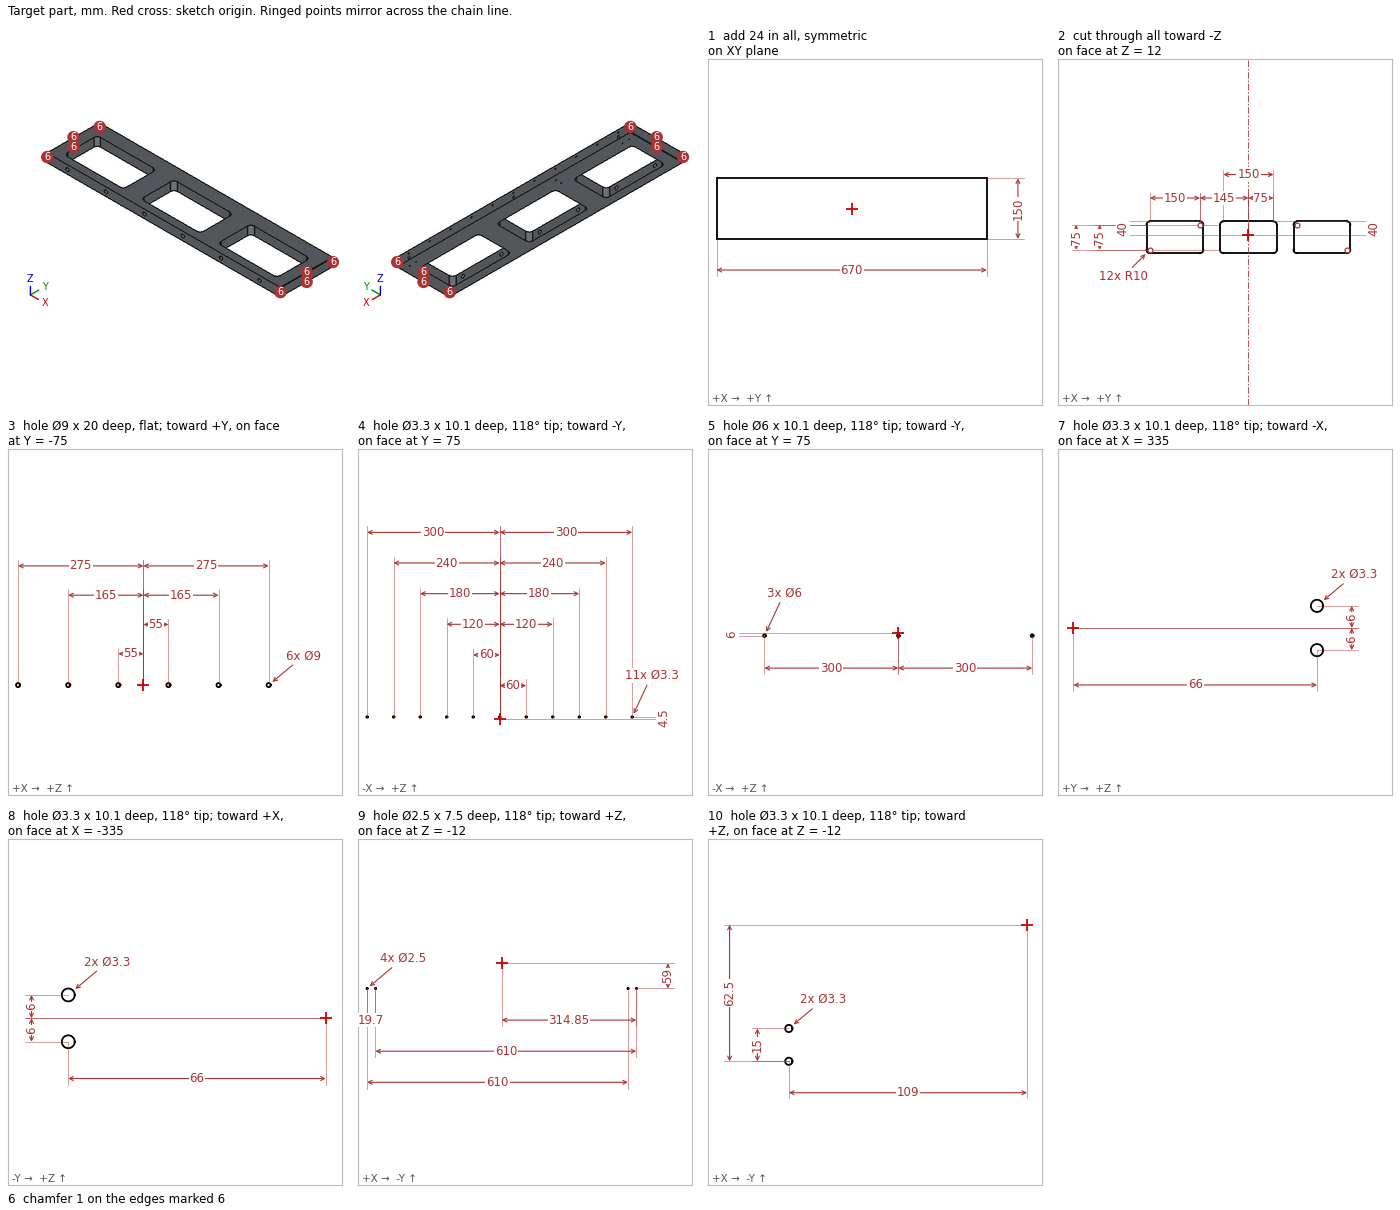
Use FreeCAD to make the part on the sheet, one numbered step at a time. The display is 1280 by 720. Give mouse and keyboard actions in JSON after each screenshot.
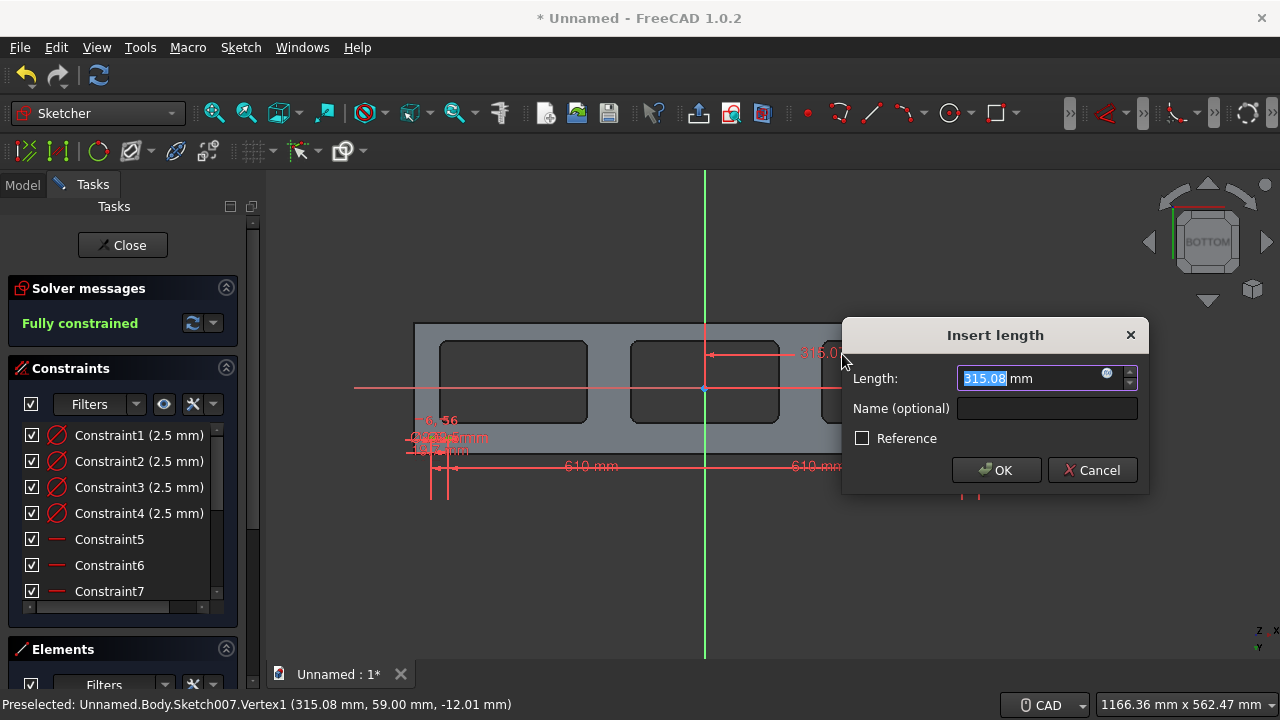
{"action": "type", "text": "314.85"}
{"action": "key", "text": "Return"}
{"action": "key", "text": "Escape"}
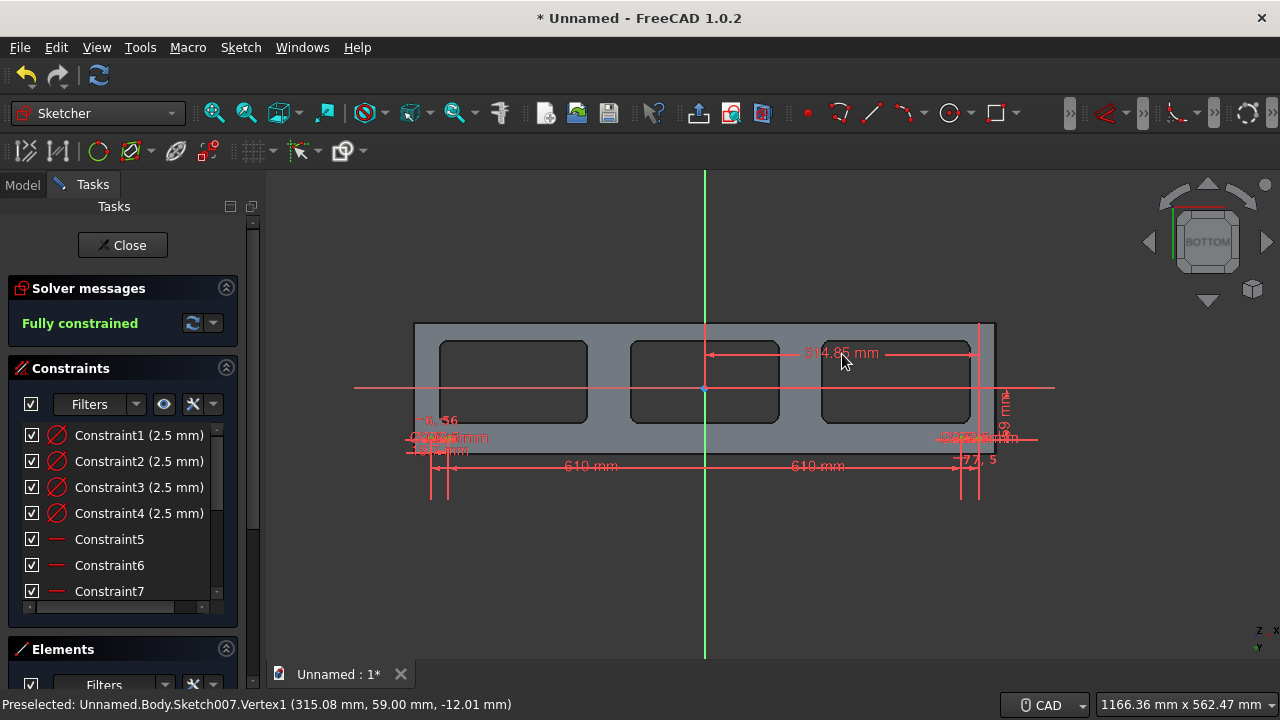
{"action": "left_click", "coordinate": [123, 245]}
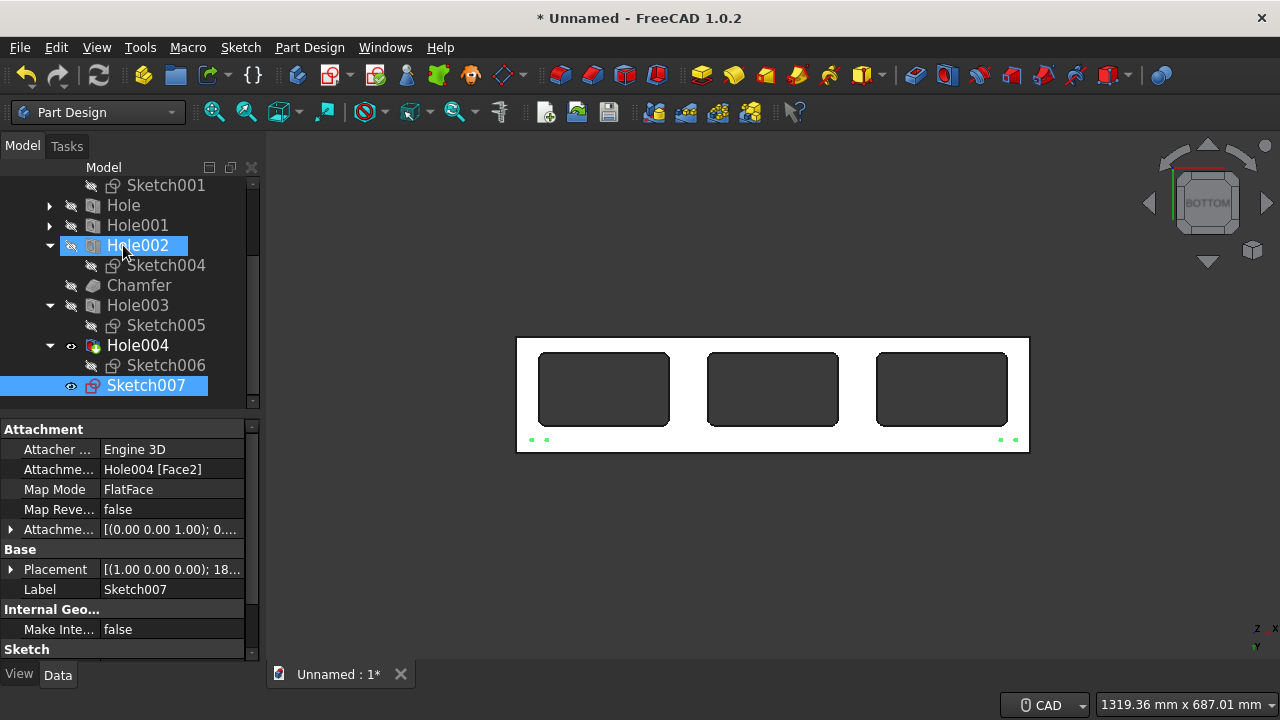
{"action": "left_click", "coordinate": [948, 76]}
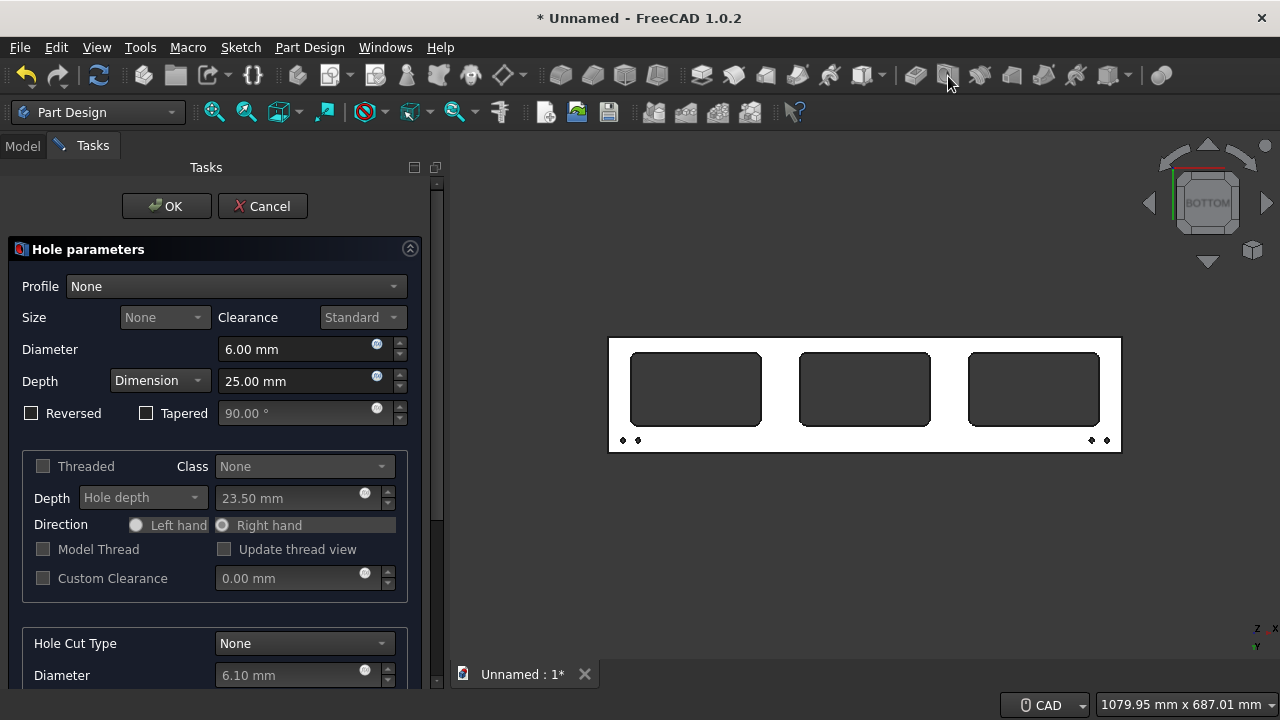
{"action": "triple_click", "coordinate": [305, 349]}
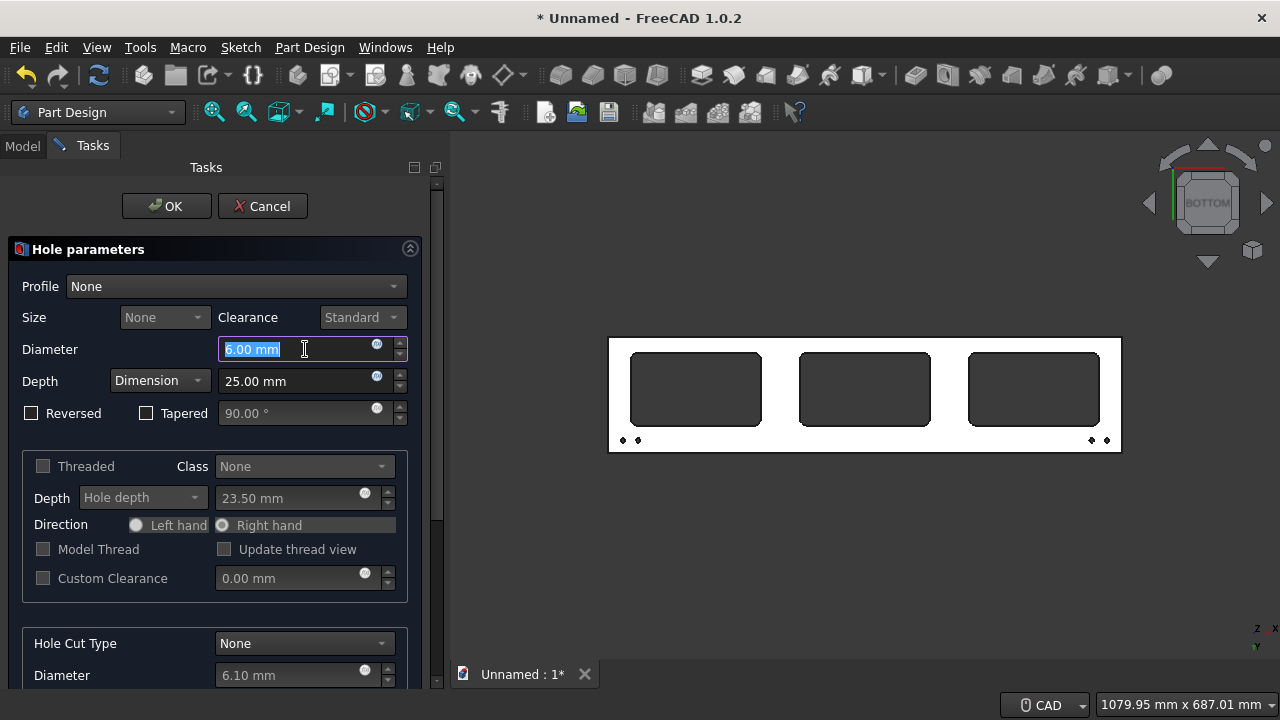
{"action": "type", "text": "2.5"}
{"action": "key", "text": "Tab"}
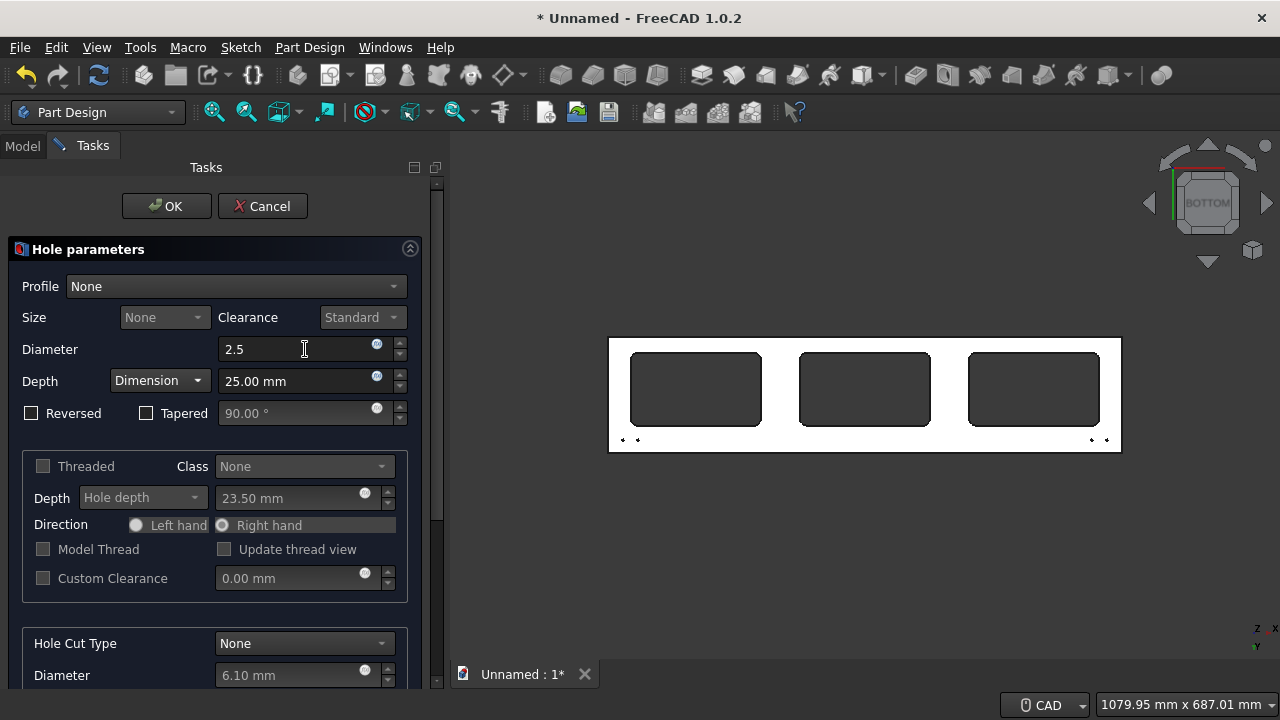
{"action": "triple_click", "coordinate": [305, 381]}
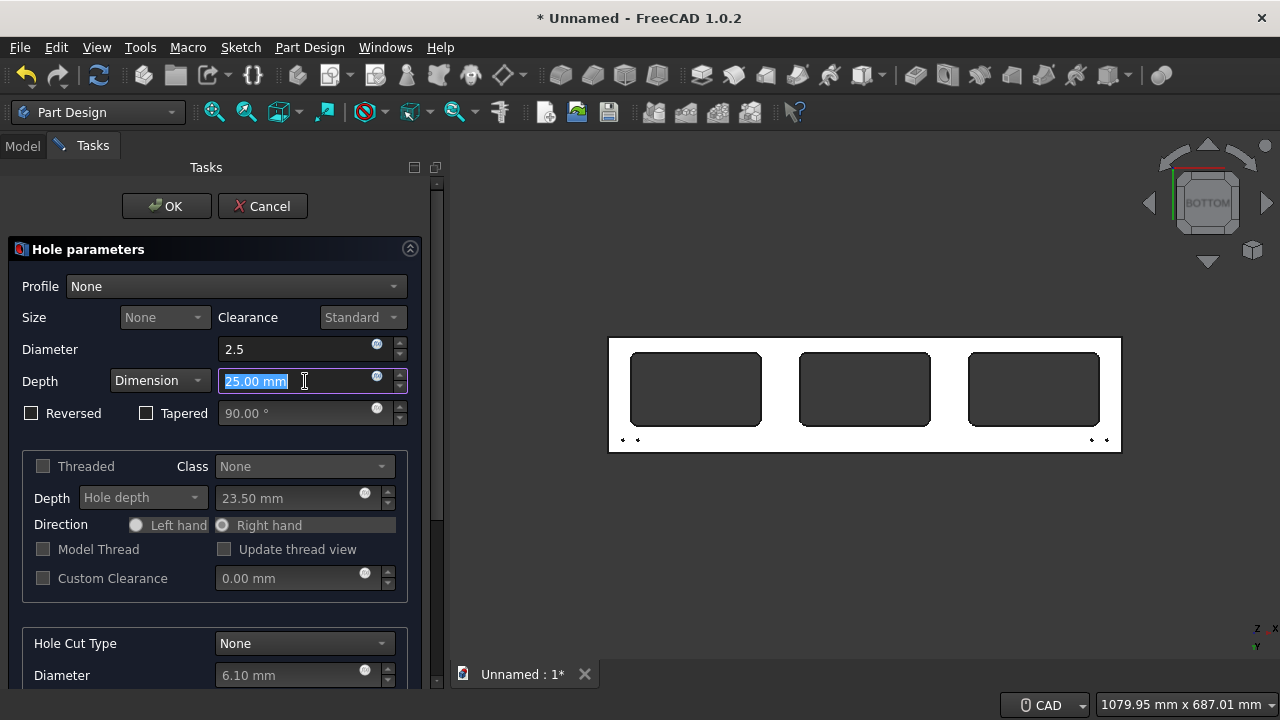
{"action": "type", "text": "7.5"}
{"action": "key", "text": "Tab"}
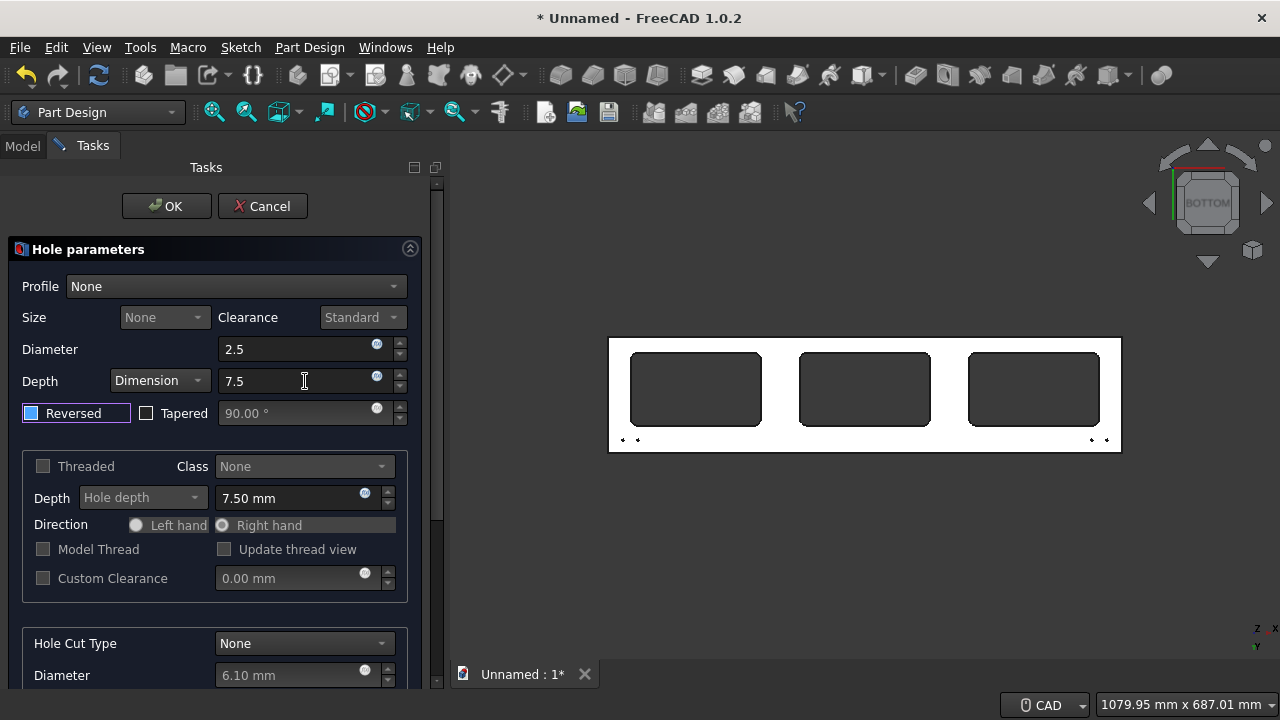
{"action": "left_click", "coordinate": [167, 206]}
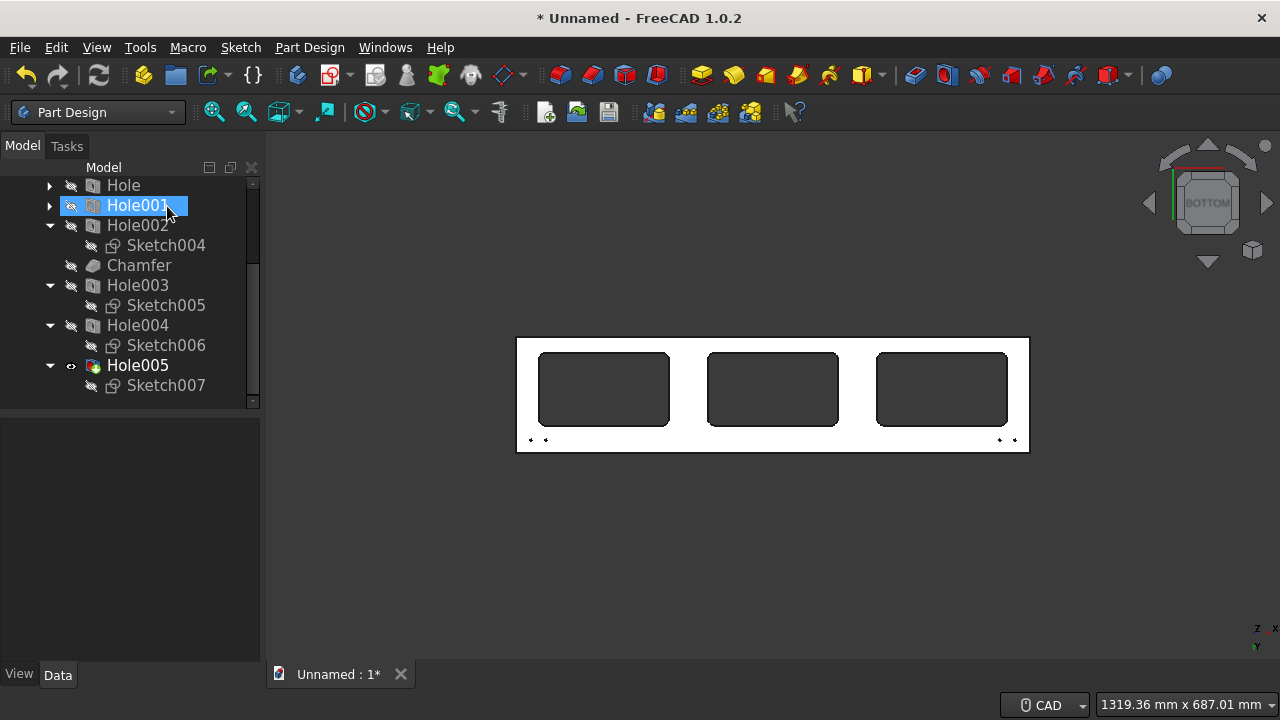
{"action": "left_click", "coordinate": [846, 427]}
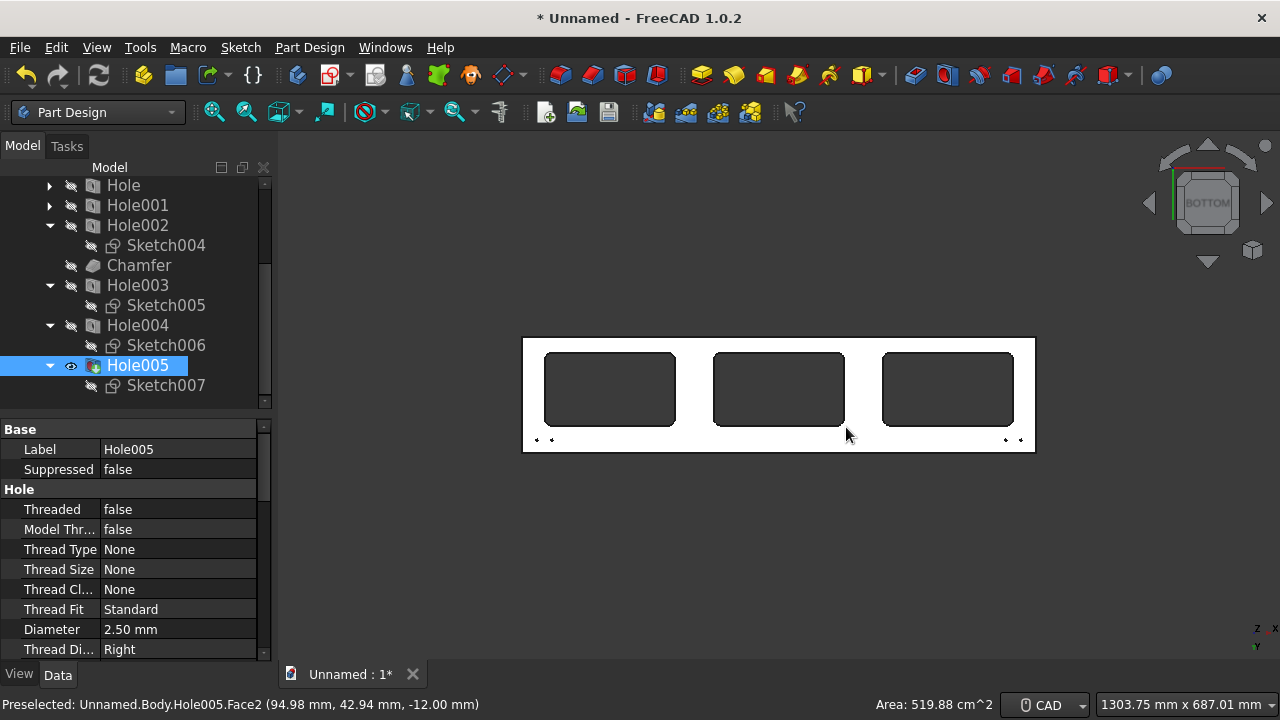
{"action": "left_click", "coordinate": [330, 76]}